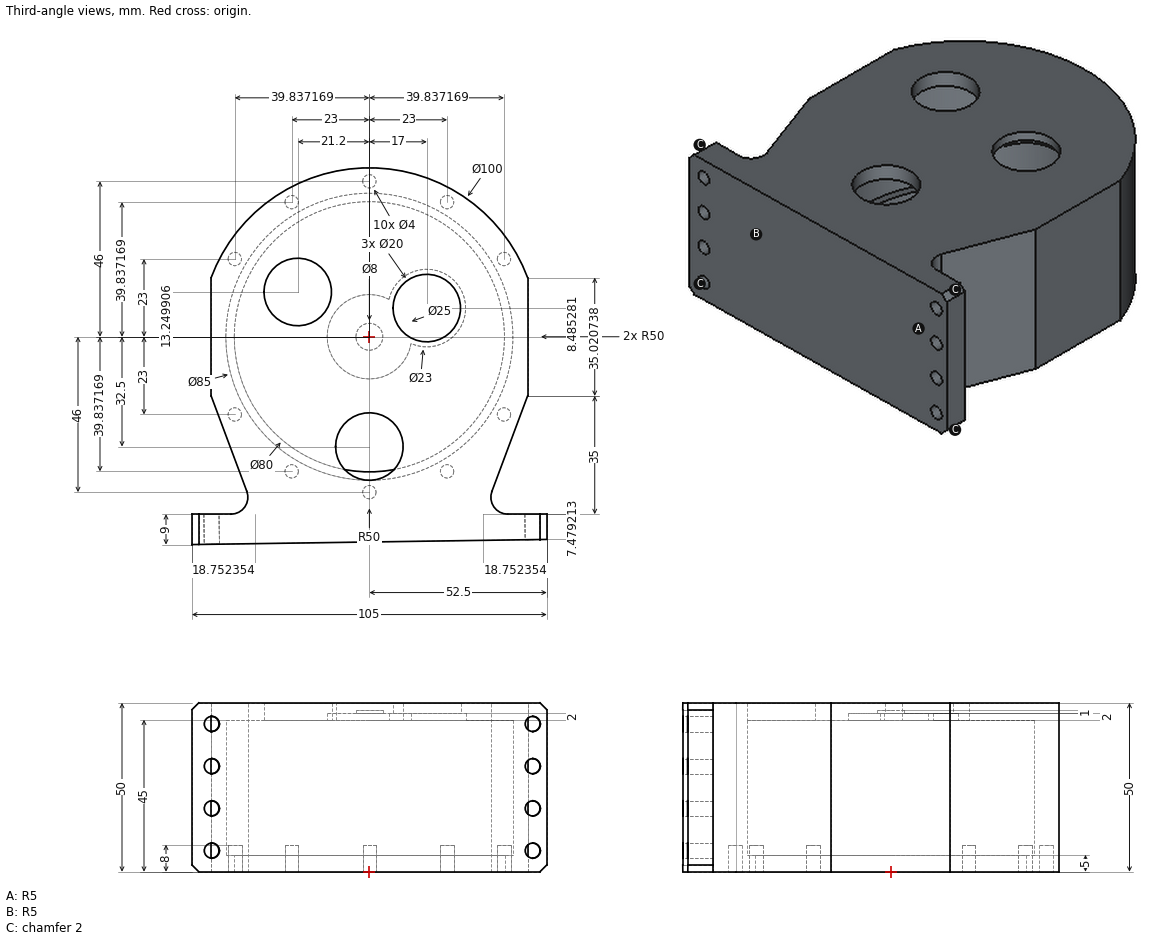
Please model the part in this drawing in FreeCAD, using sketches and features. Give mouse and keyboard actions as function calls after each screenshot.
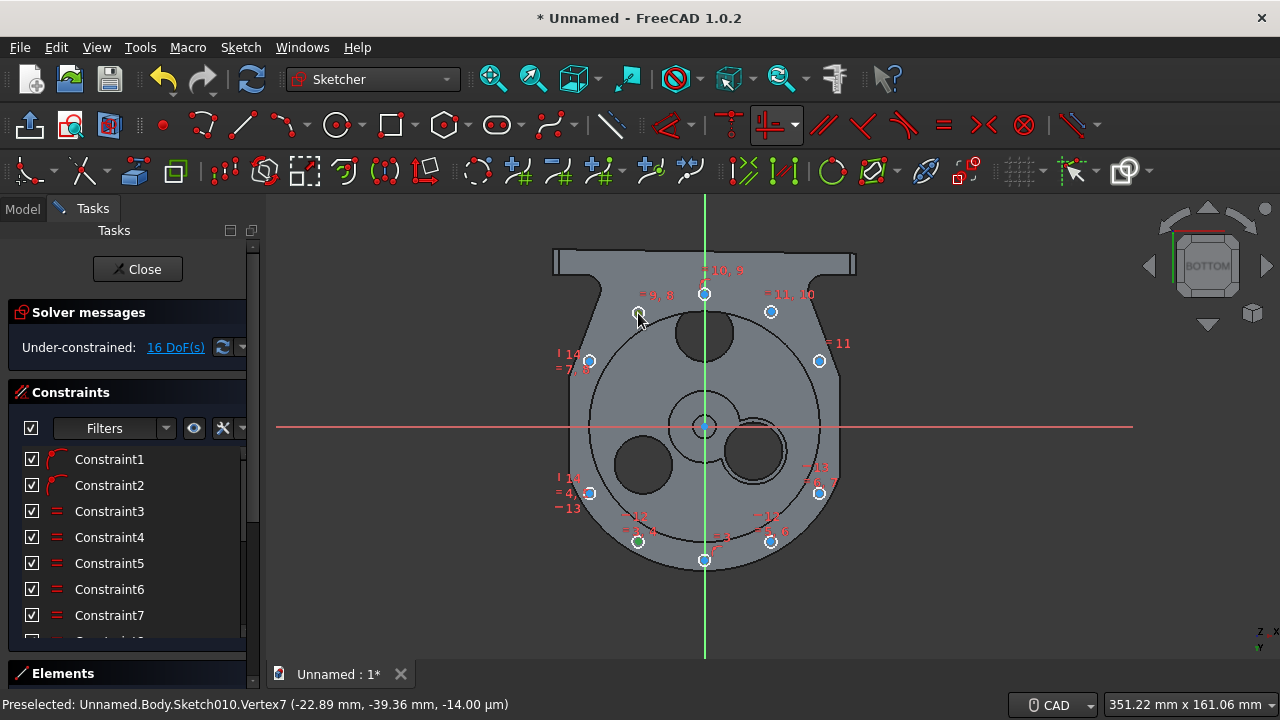
key(v)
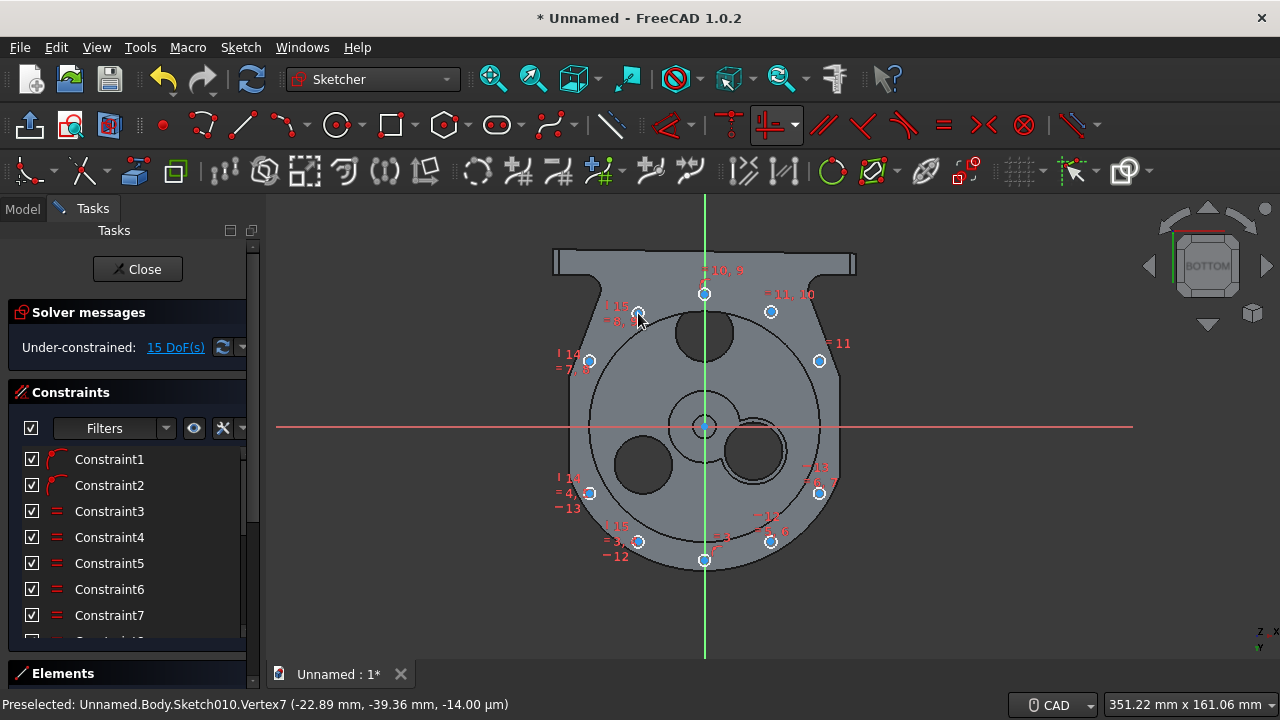
click(771, 542)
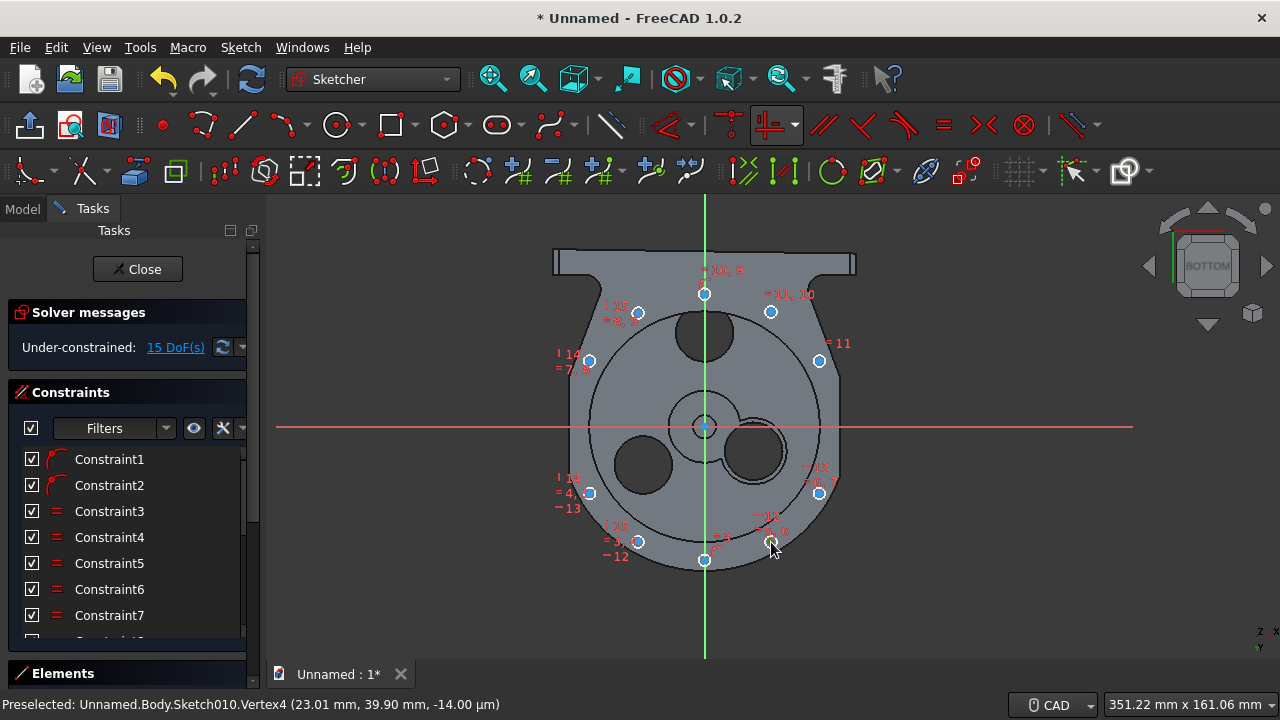
click(771, 312)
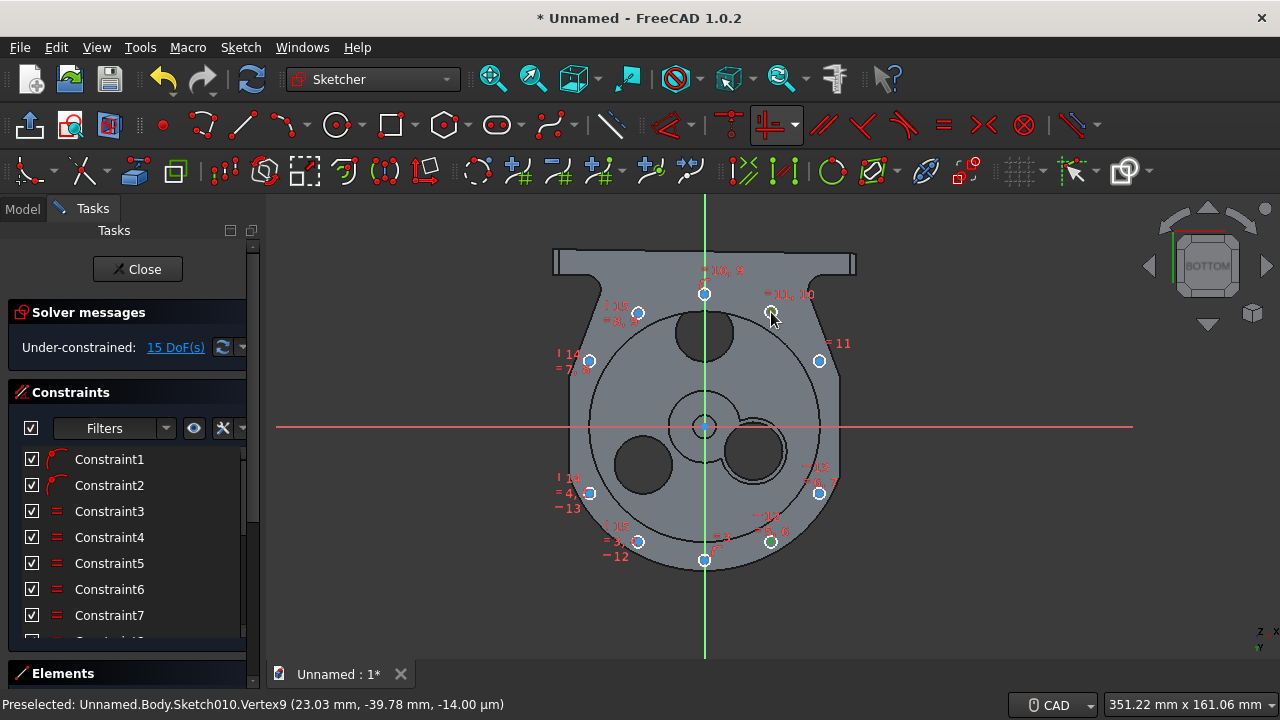
click(798, 126)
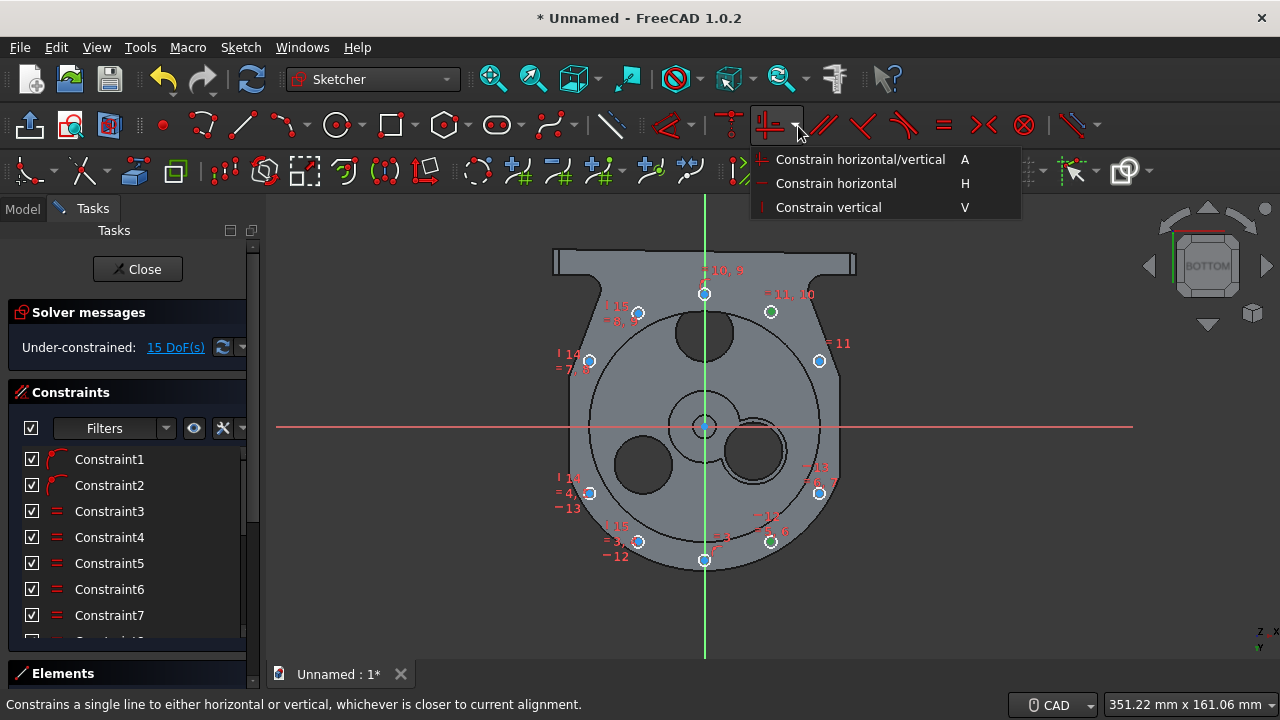
click(886, 207)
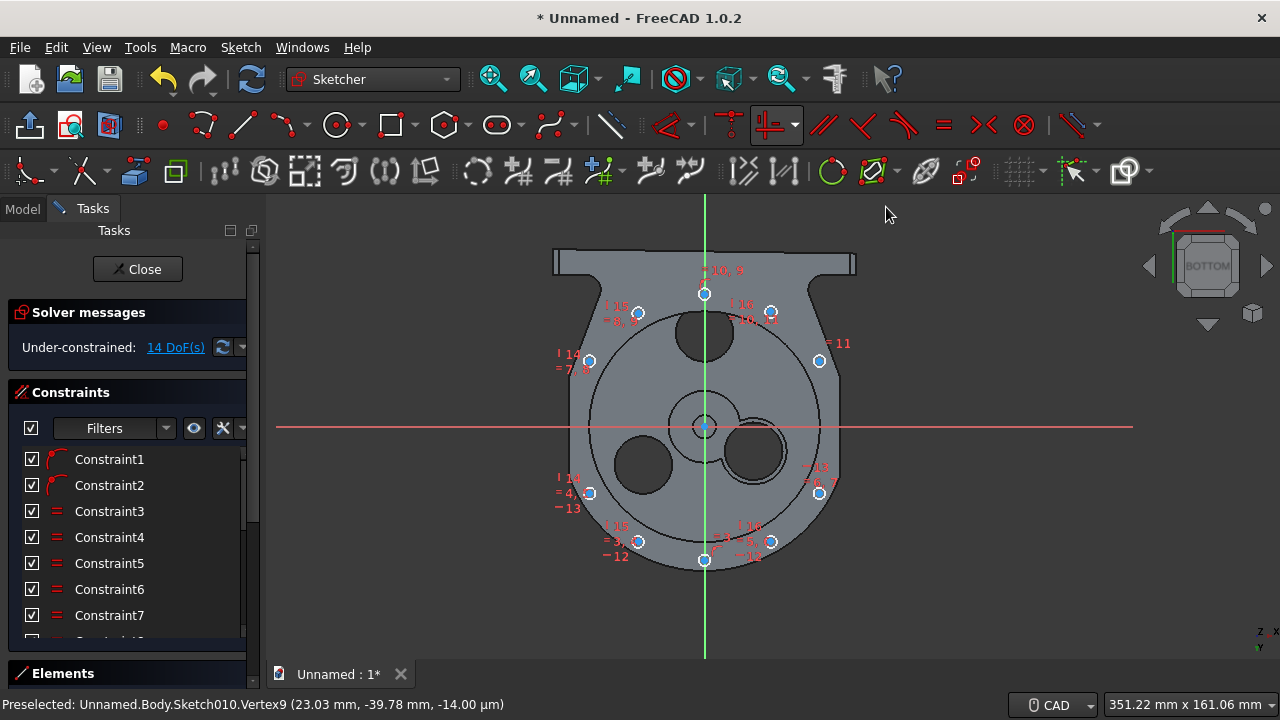
click(640, 315)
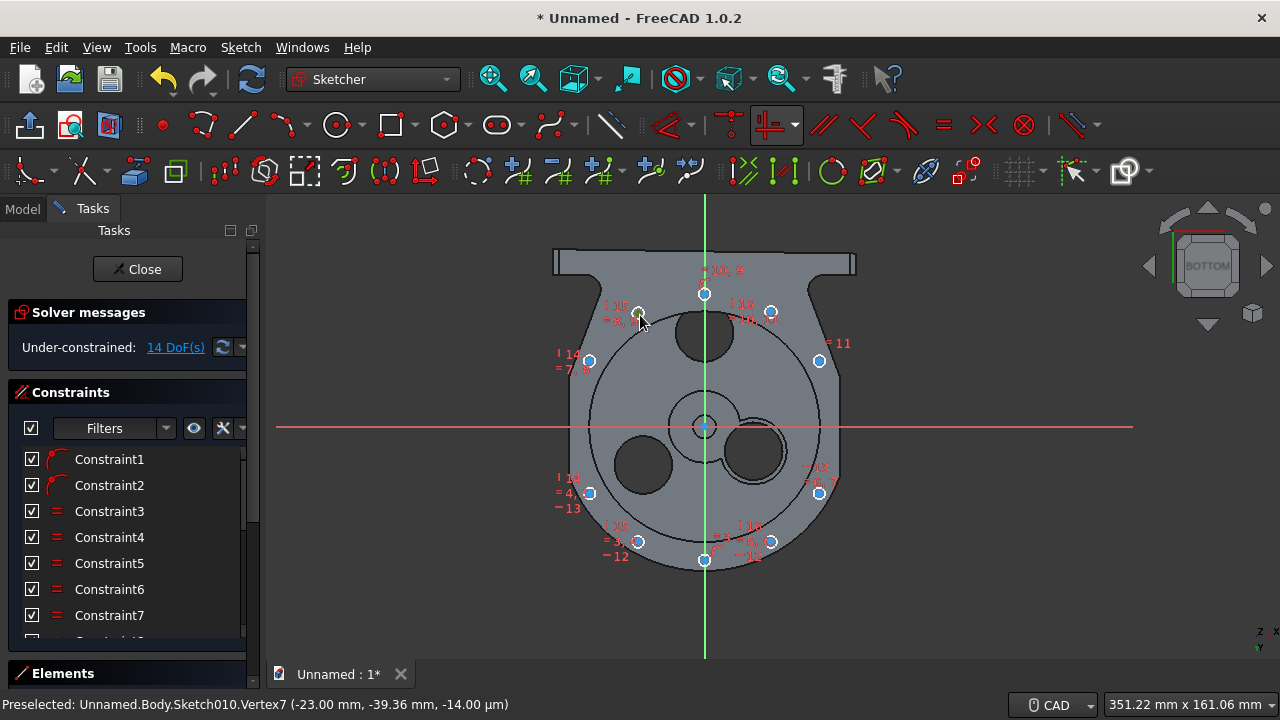
scroll(771, 312, up, 4)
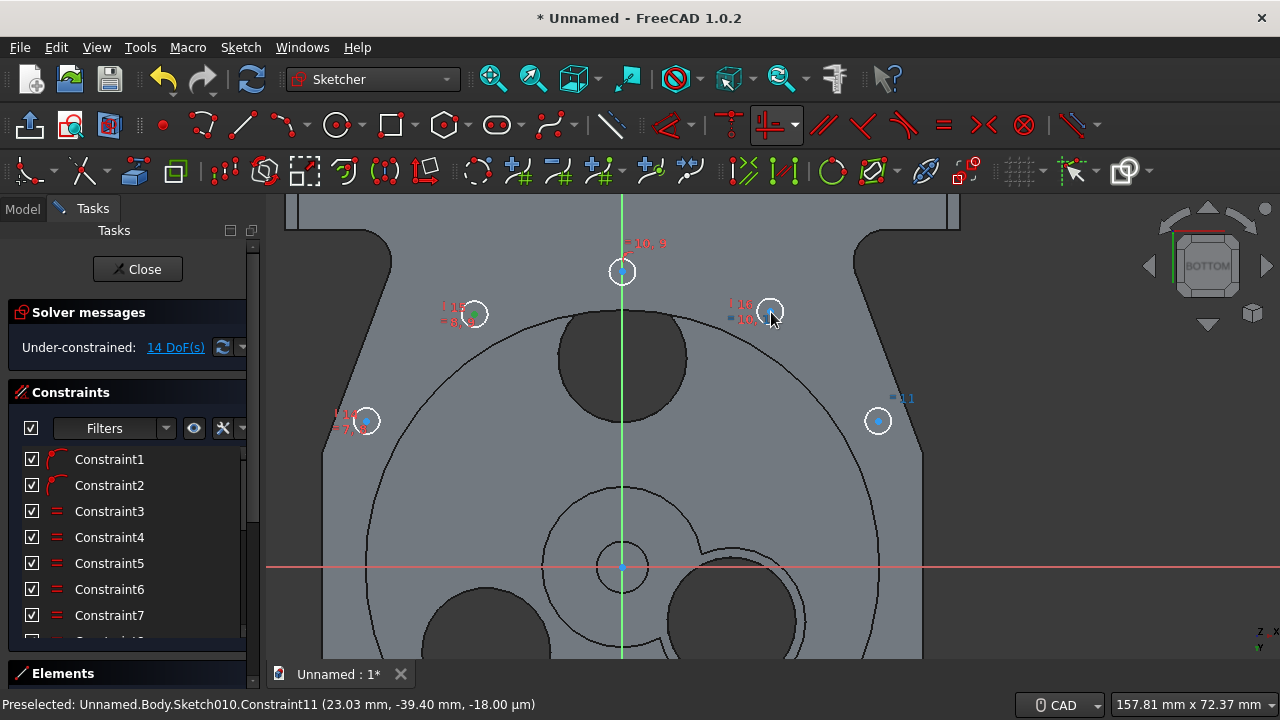
scroll(770, 311, up, 4)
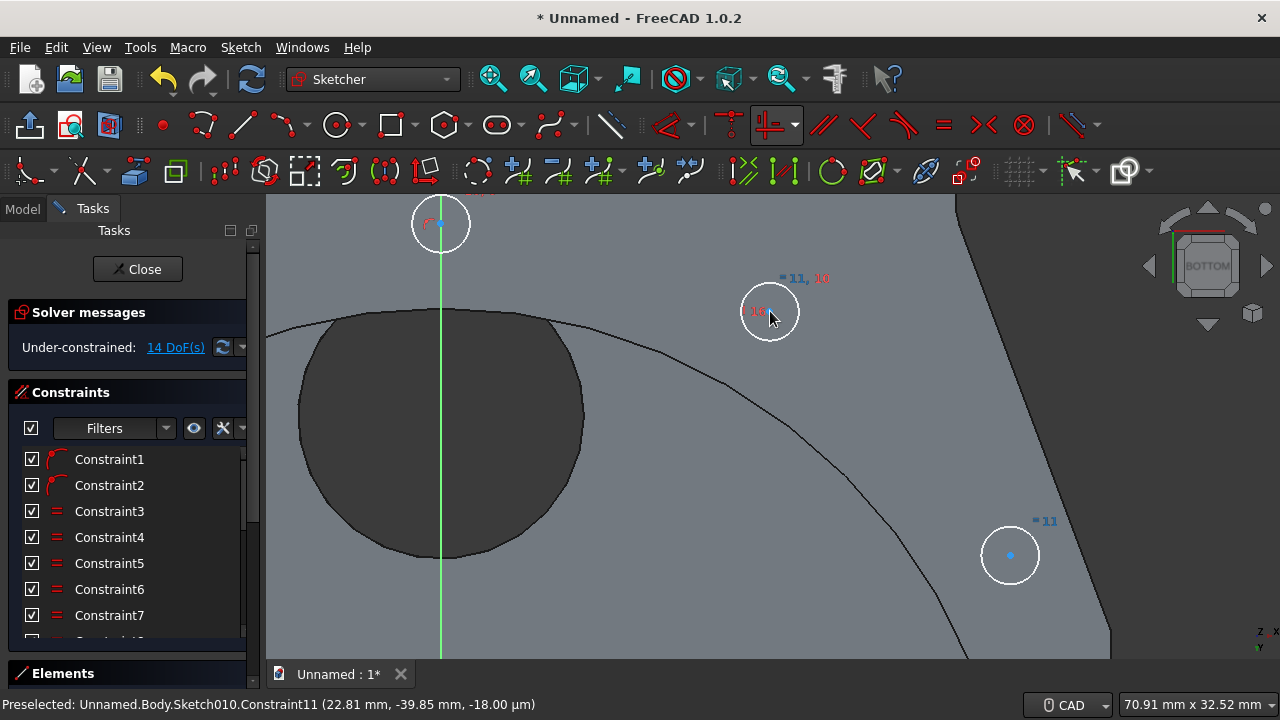
click(770, 312)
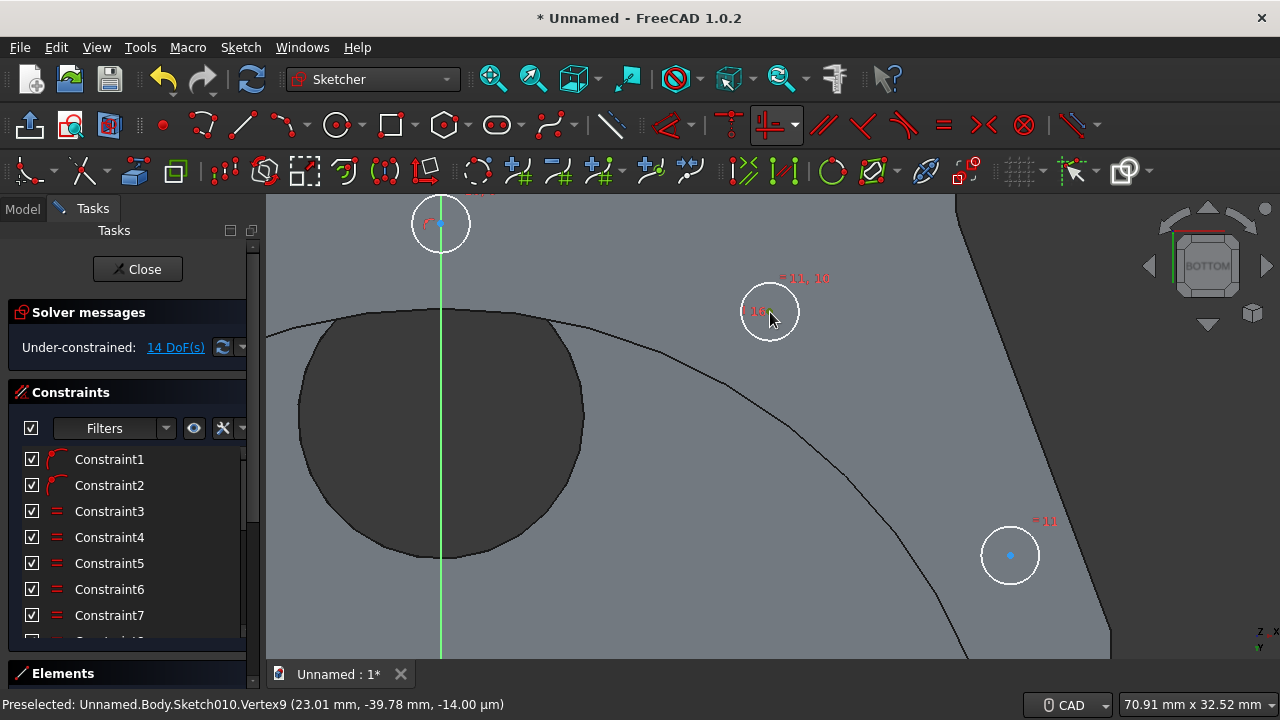
click(798, 126)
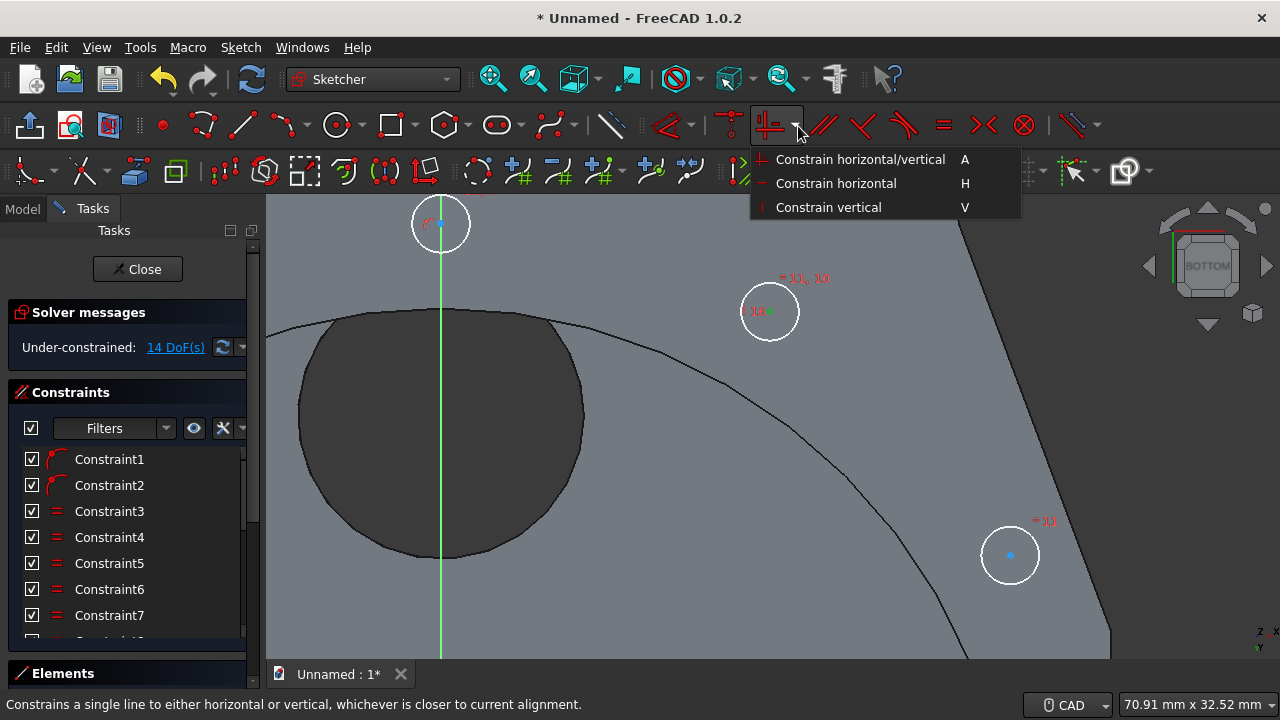
click(886, 183)